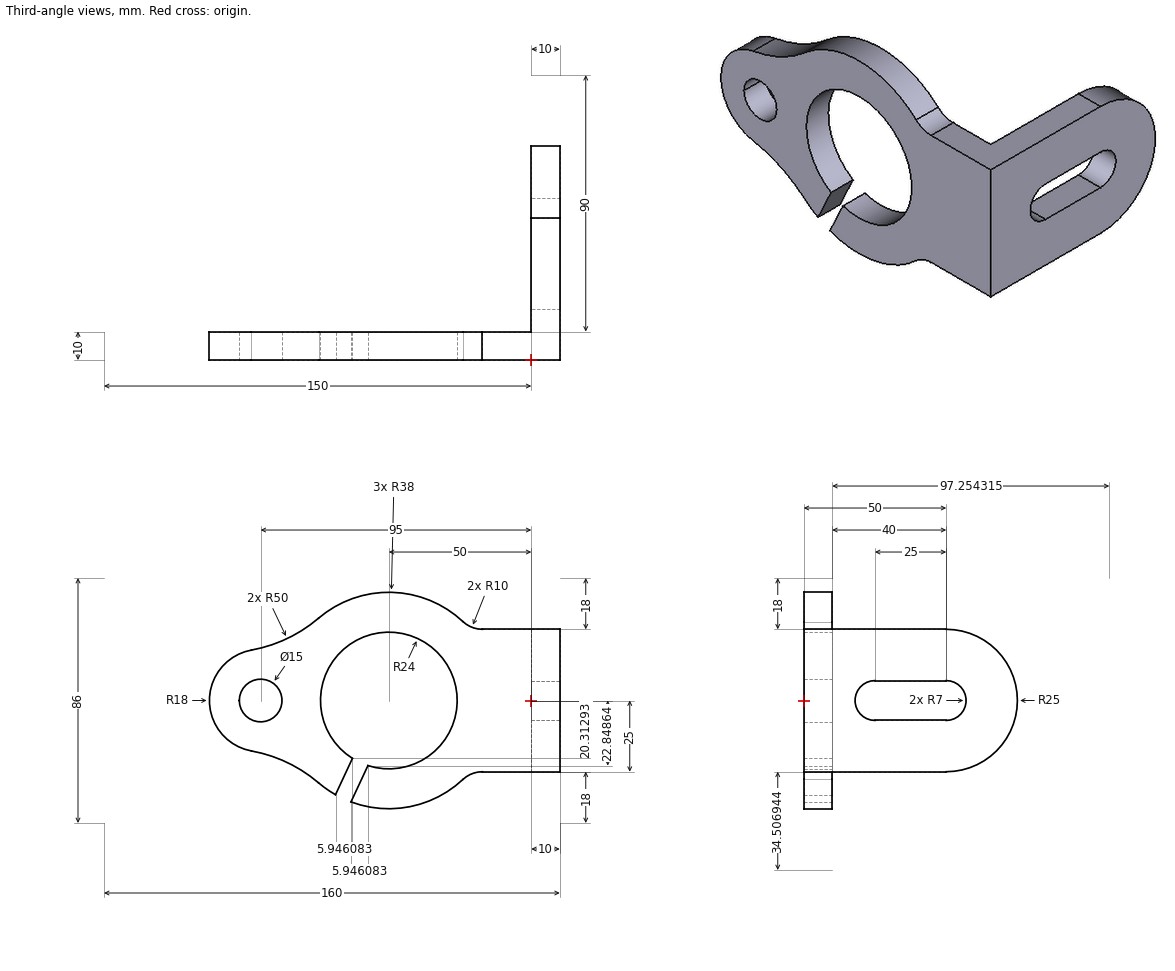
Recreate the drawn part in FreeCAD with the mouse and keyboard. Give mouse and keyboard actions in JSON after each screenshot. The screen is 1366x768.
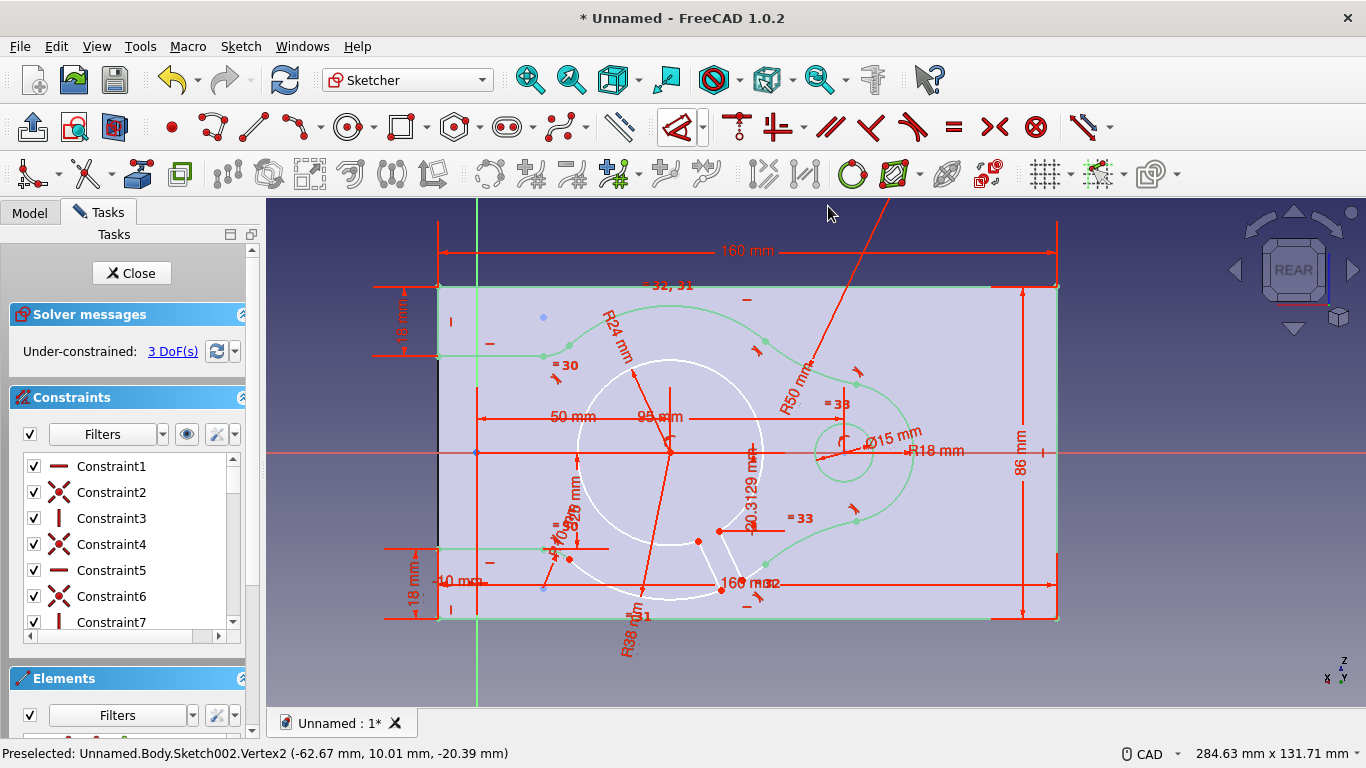
{"action": "left_click", "coordinate": [698, 541]}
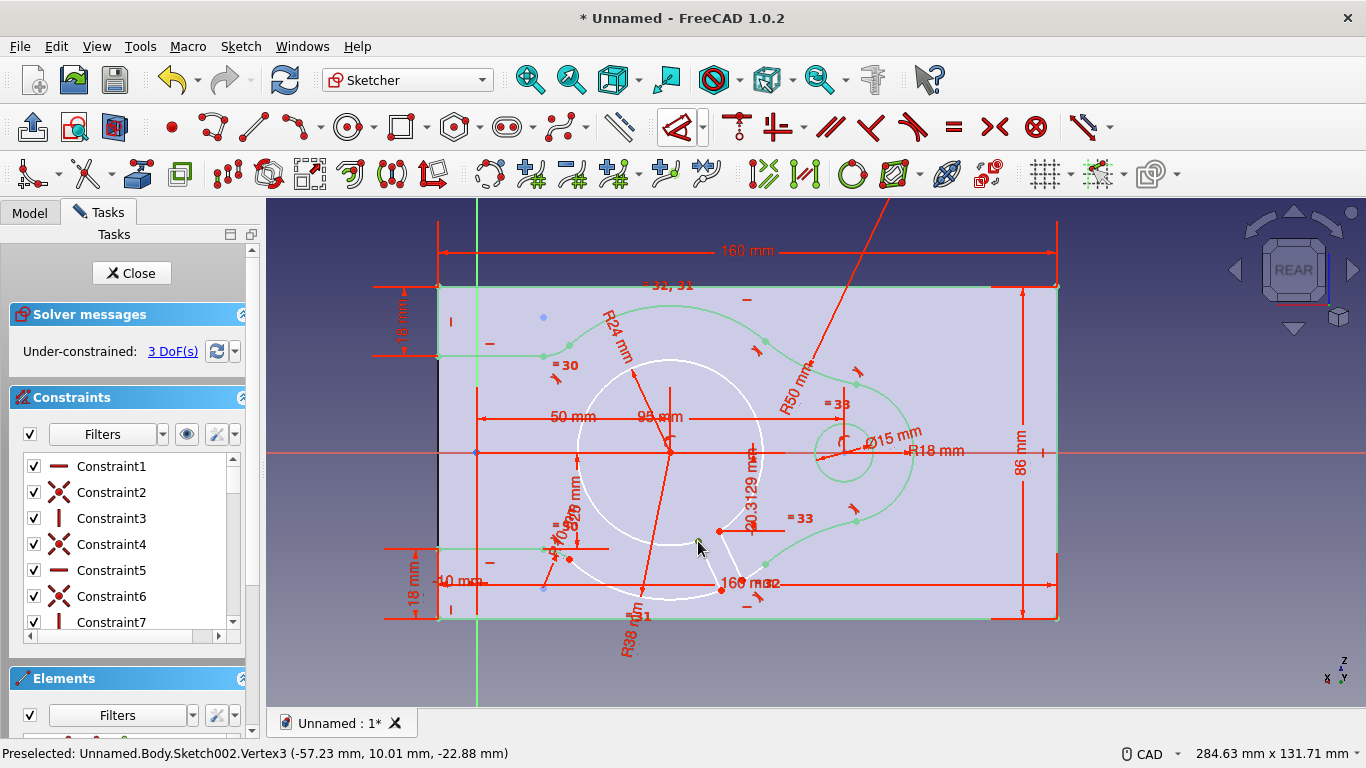
{"action": "key", "text": "i"}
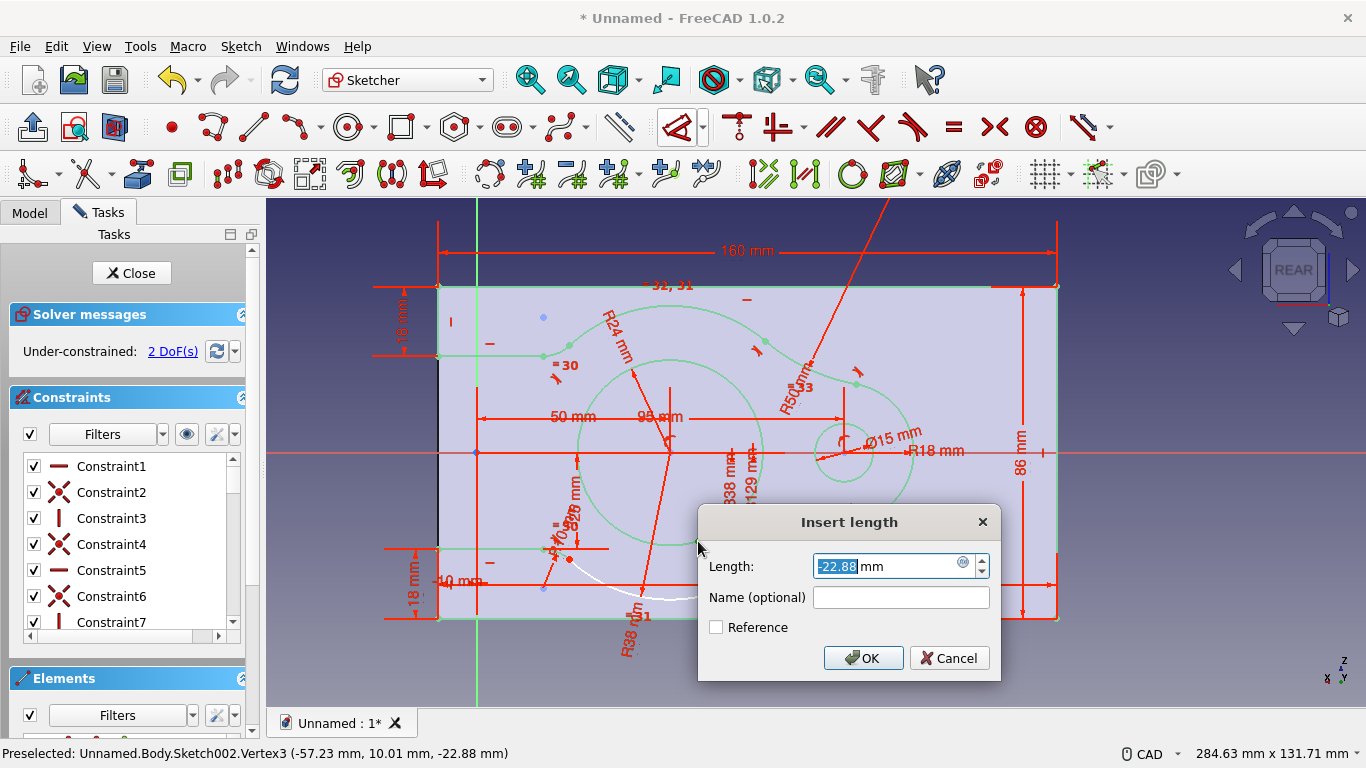
{"action": "type", "text": "-22.84864"}
{"action": "key", "text": "Return"}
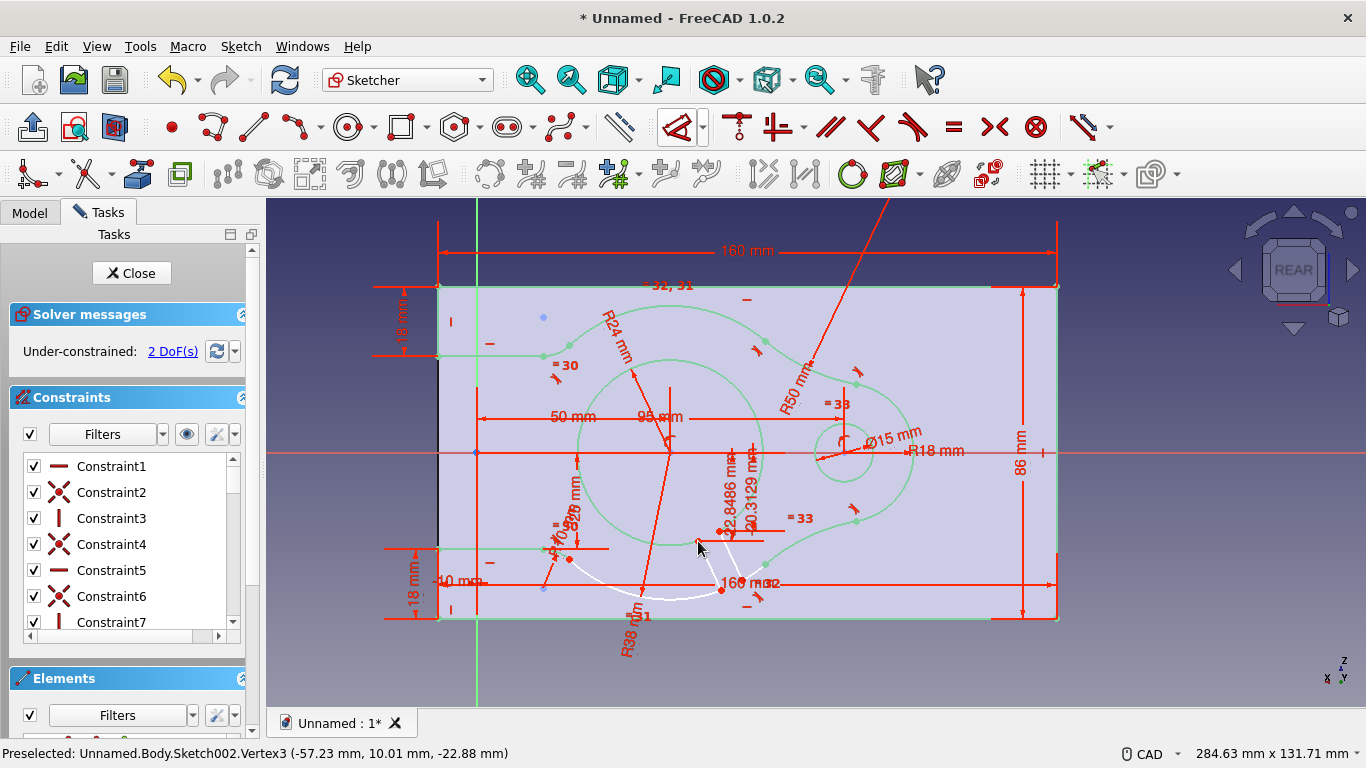
{"action": "scroll", "coordinate": [736, 566], "scroll_direction": "up", "scroll_amount": 3}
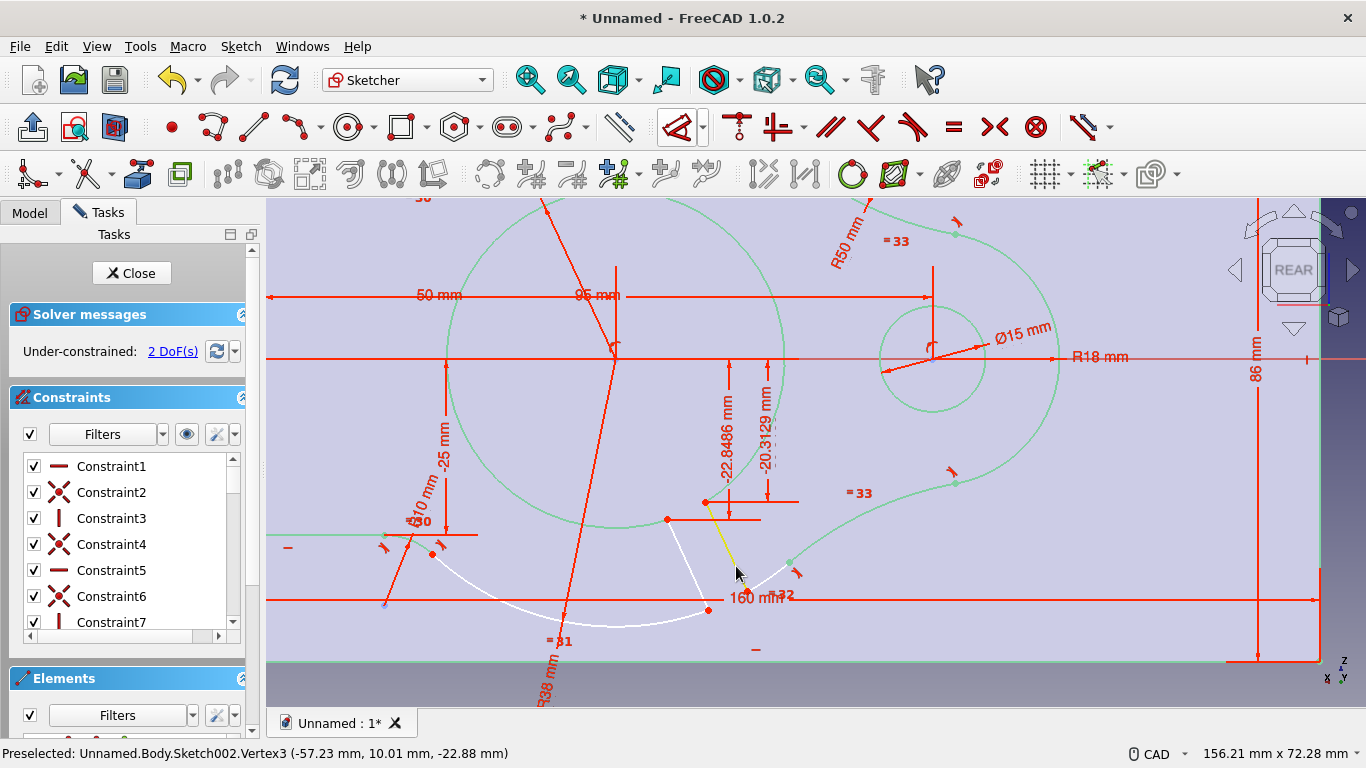
{"action": "left_click", "coordinate": [735, 565]}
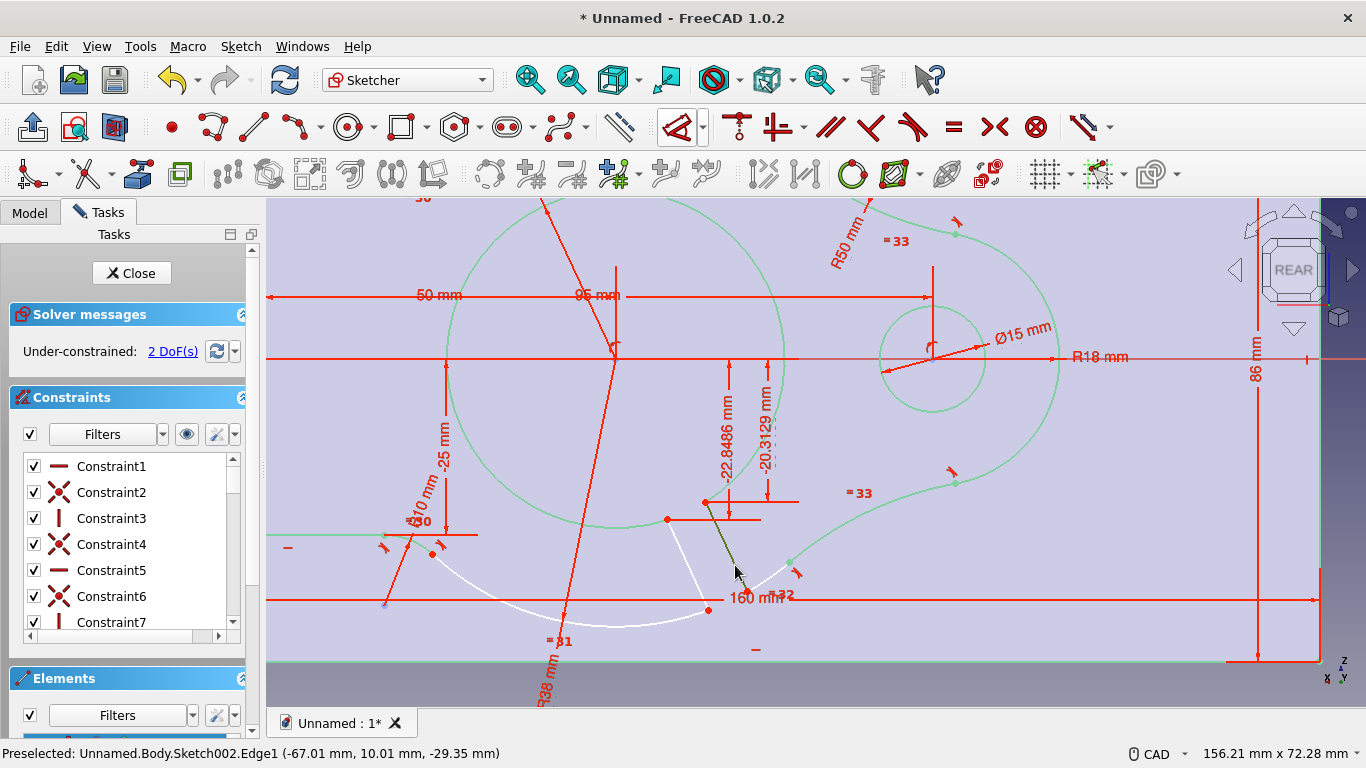
{"action": "left_click", "coordinate": [702, 128]}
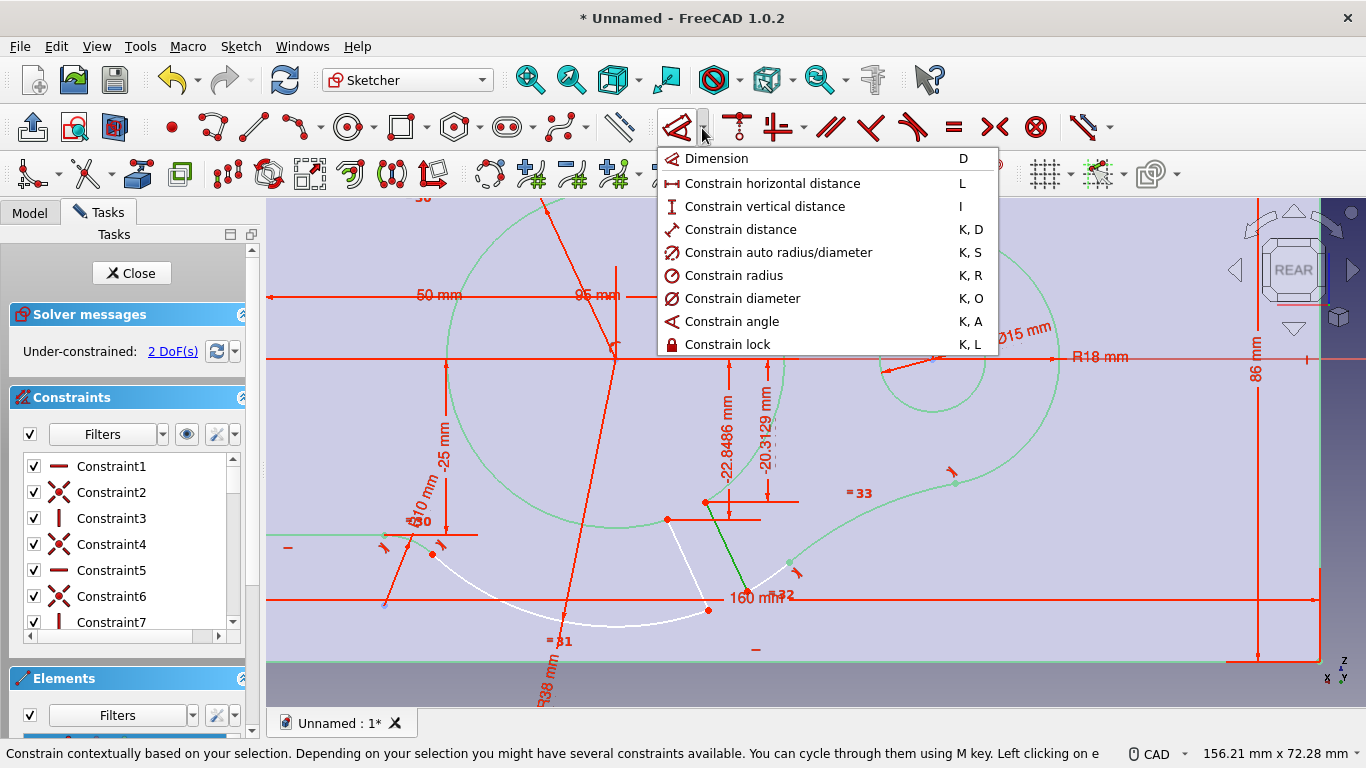
{"action": "left_click", "coordinate": [828, 184]}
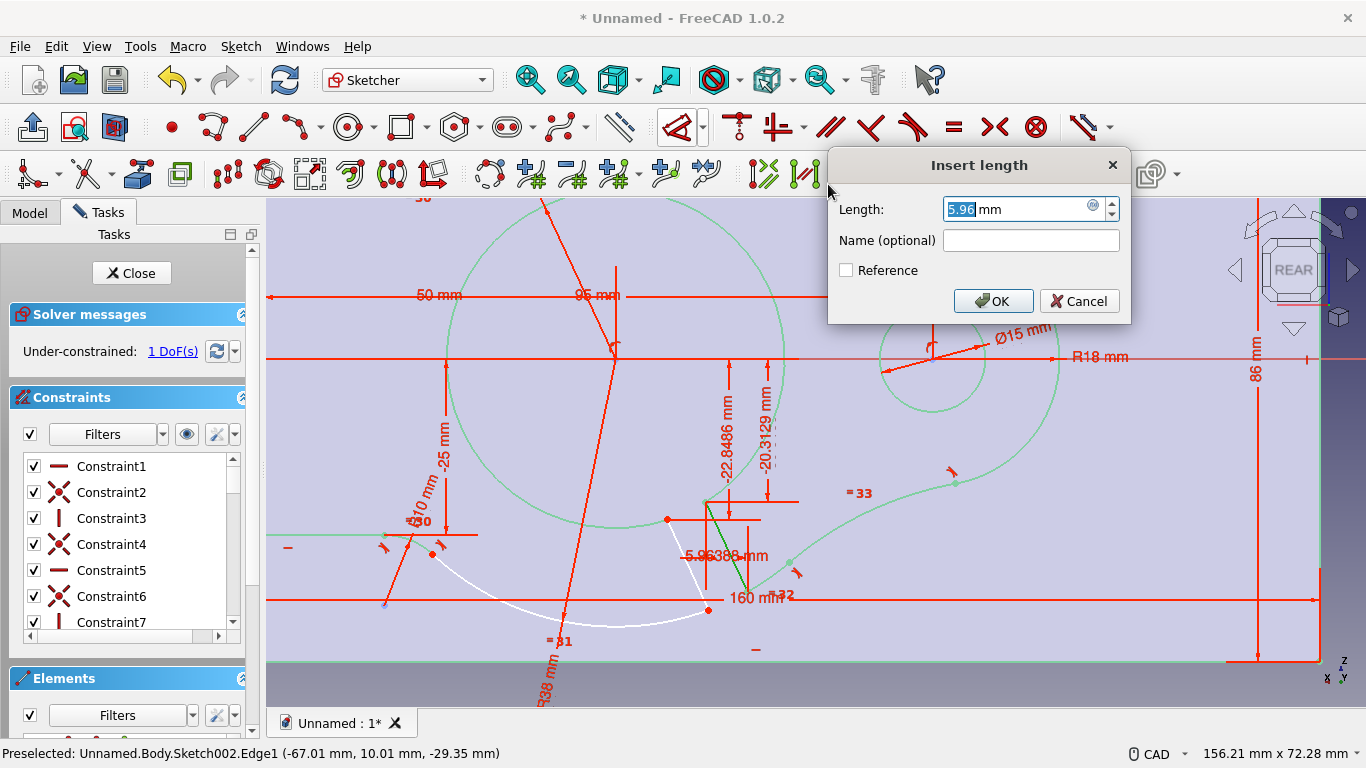
{"action": "type", "text": "5.946083"}
{"action": "key", "text": "Return"}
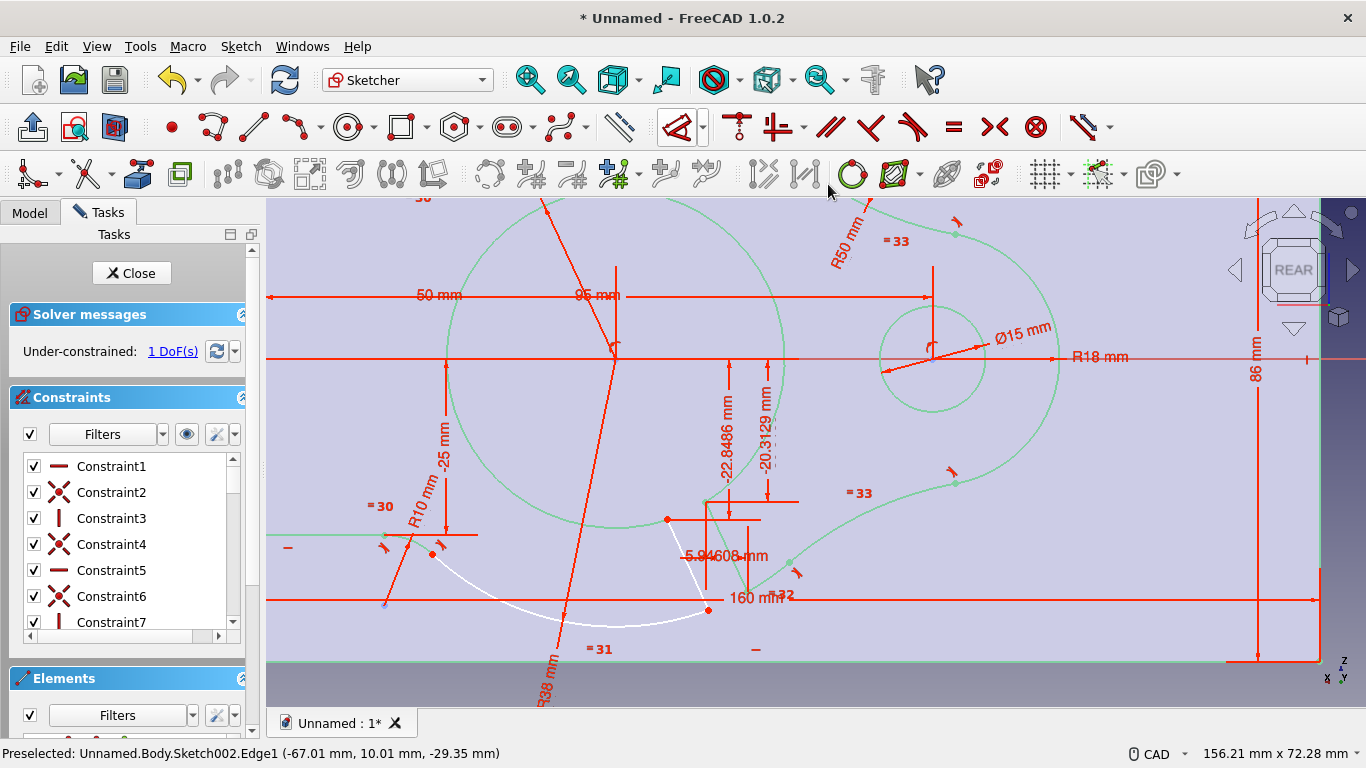
{"action": "left_click", "coordinate": [680, 547]}